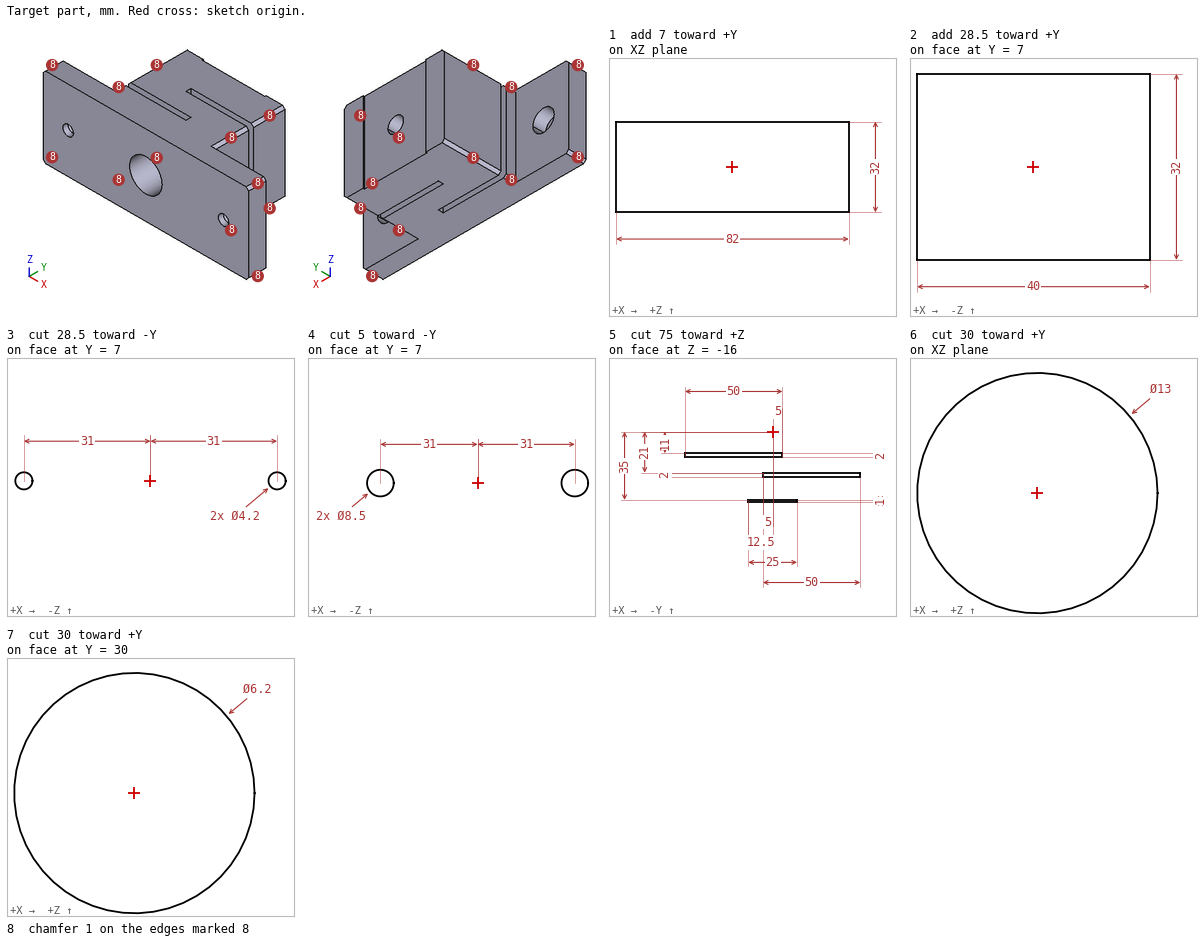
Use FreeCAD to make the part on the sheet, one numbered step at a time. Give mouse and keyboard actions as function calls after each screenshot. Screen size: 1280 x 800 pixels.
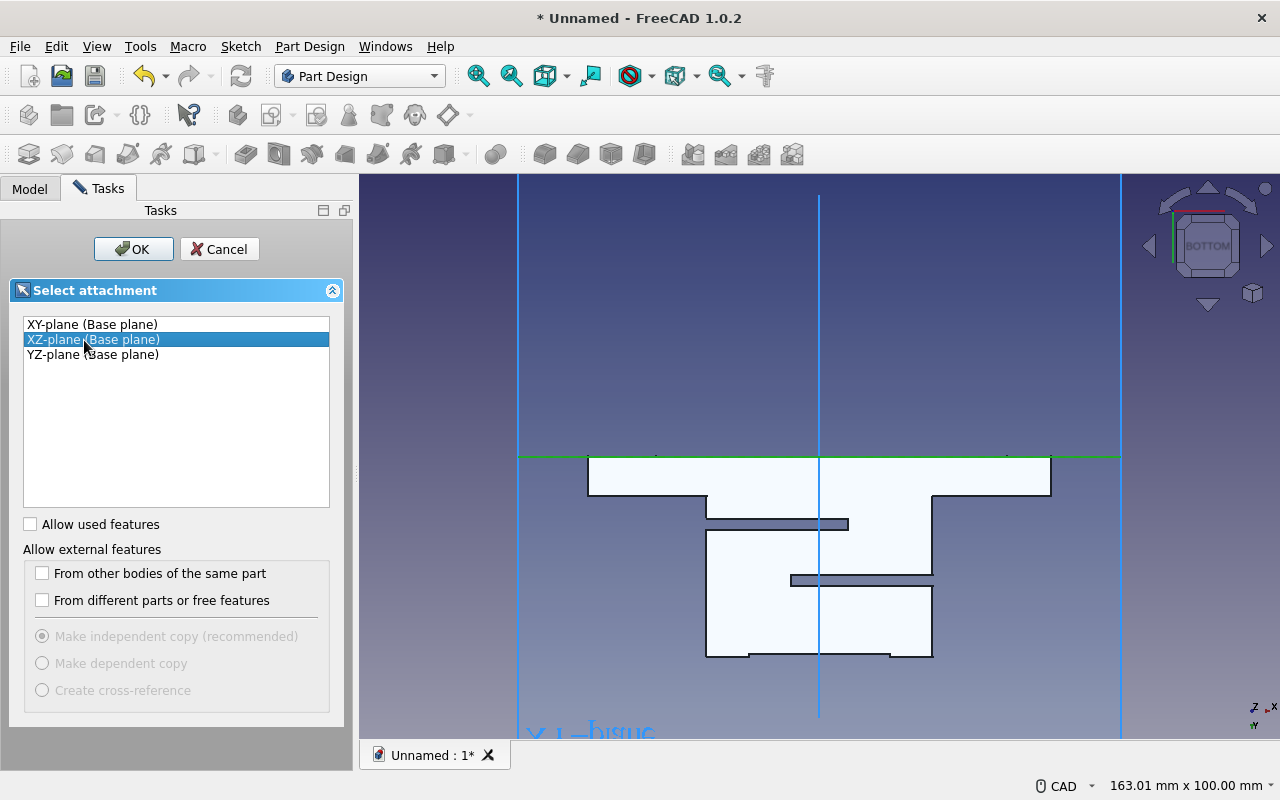
click(134, 249)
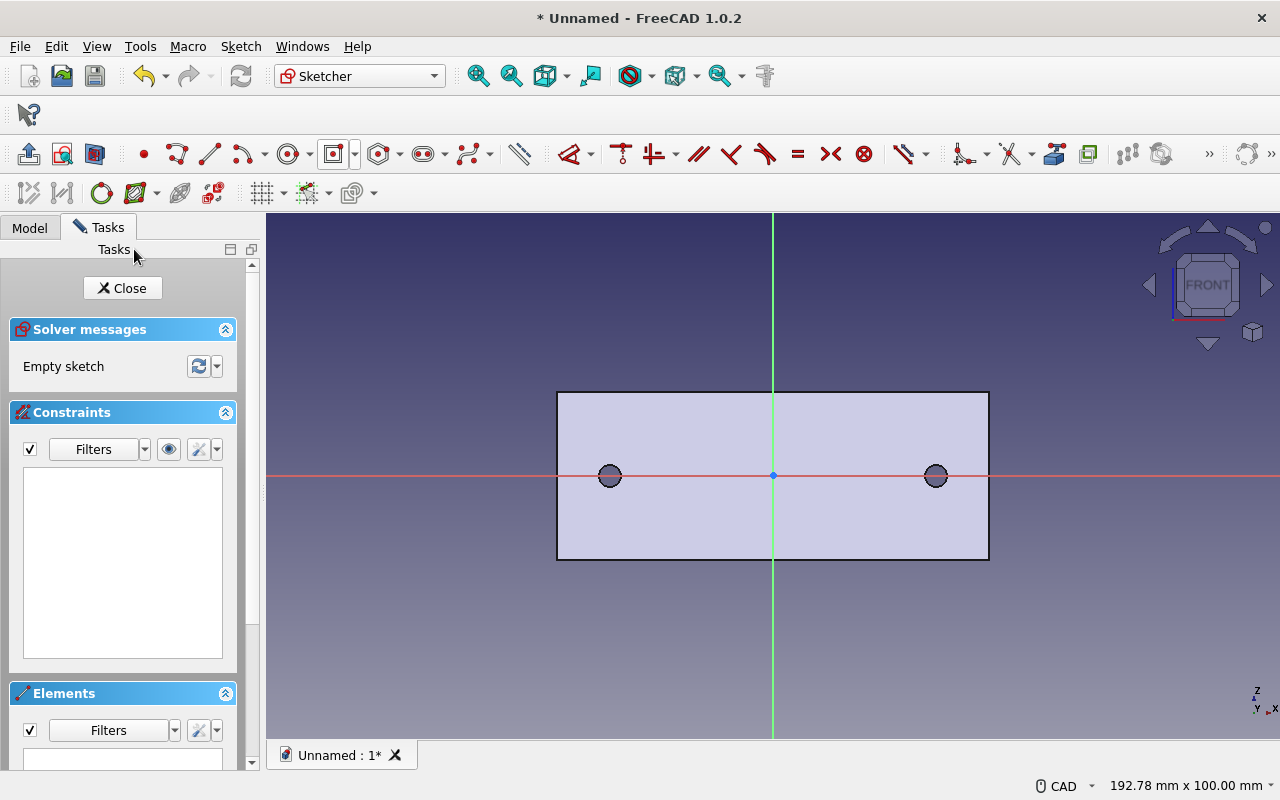
scroll(790, 476, up, 8)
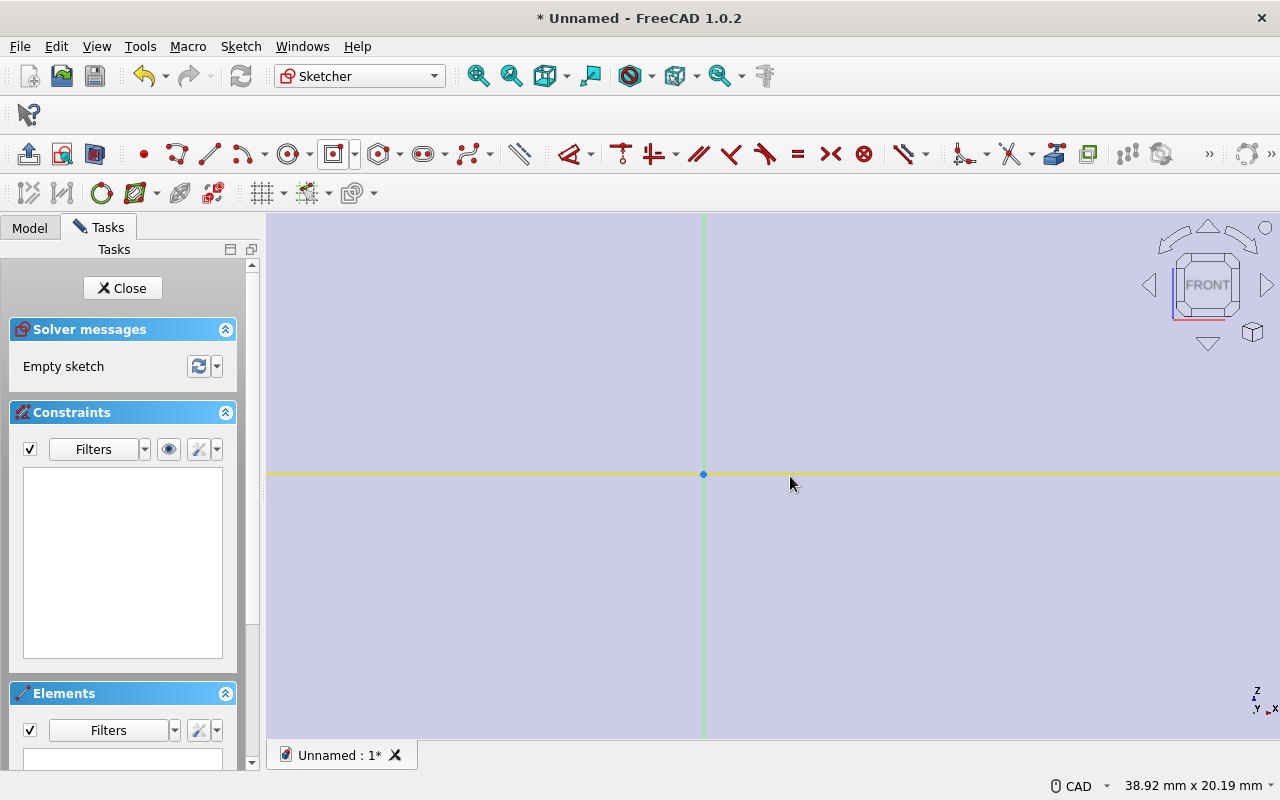
key(g)
key(c)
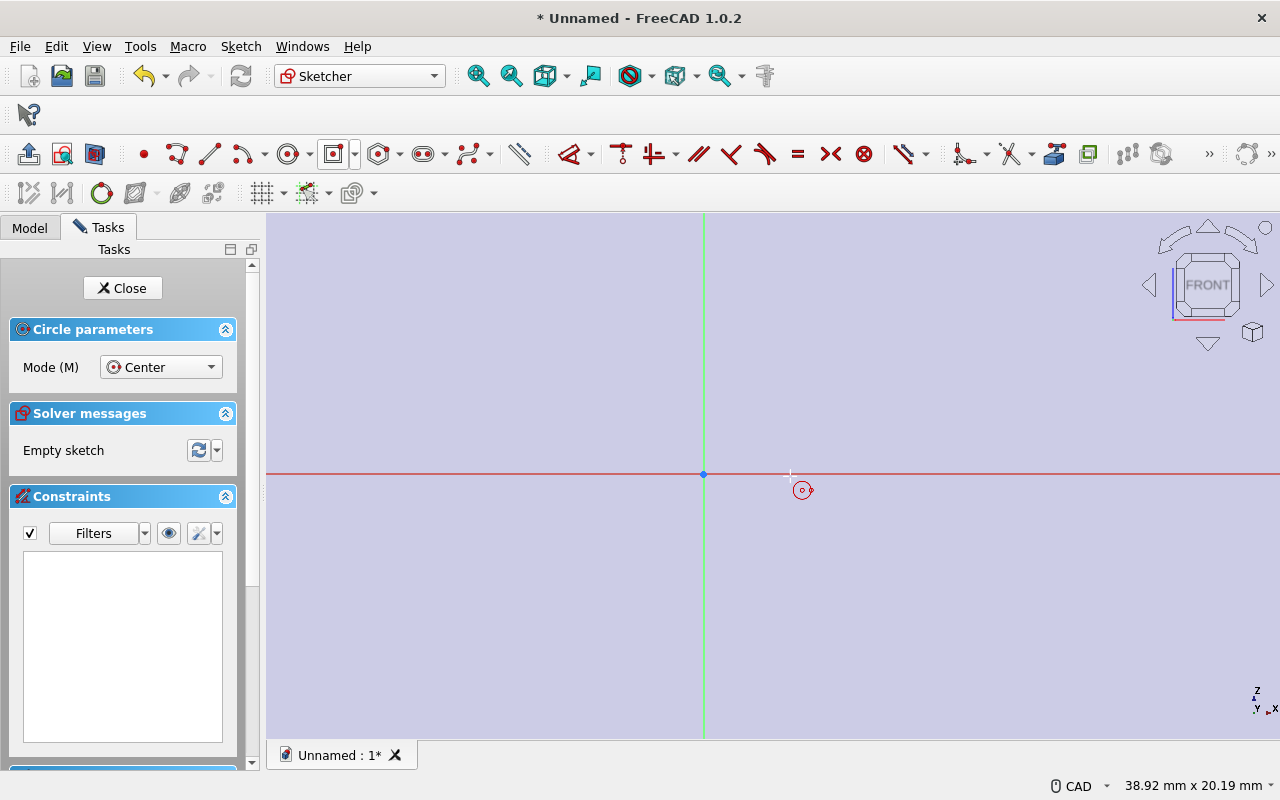
click(704, 474)
move(823, 354)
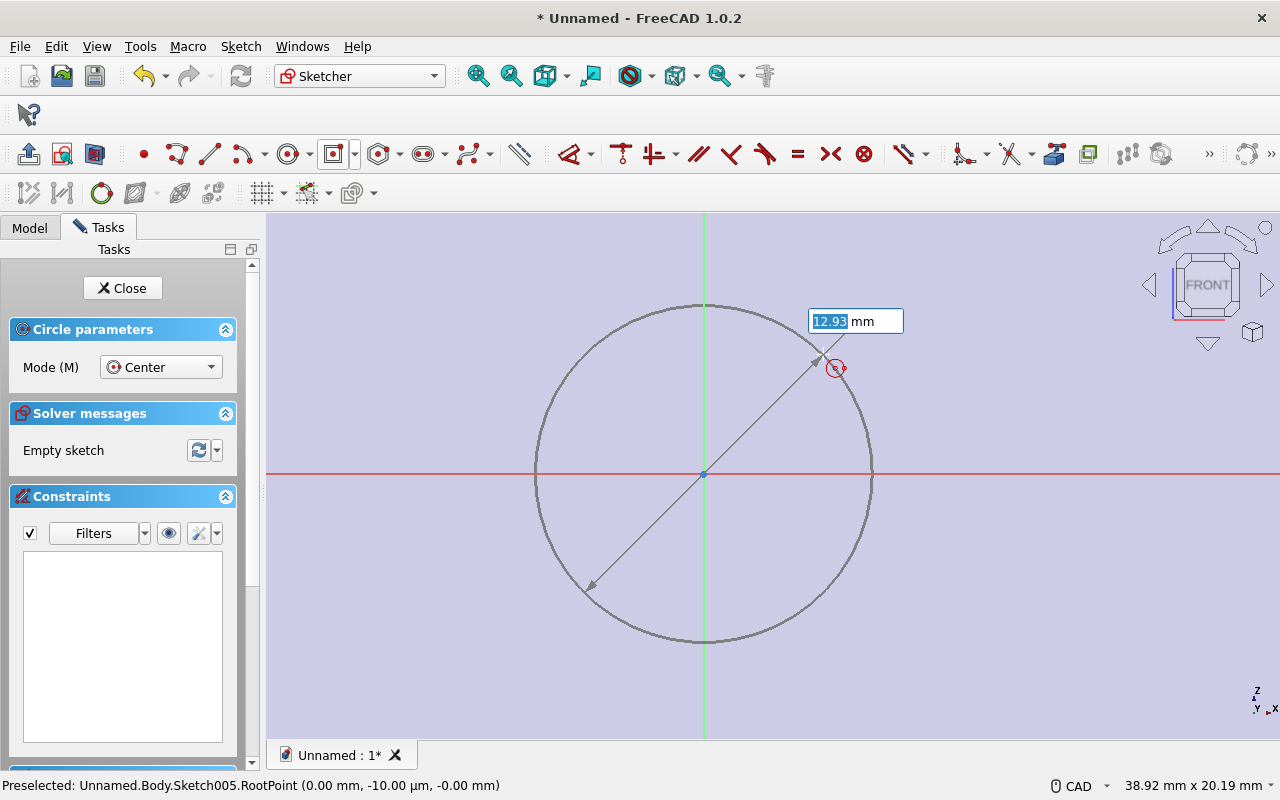
text(13)
key(Return)
key(Escape)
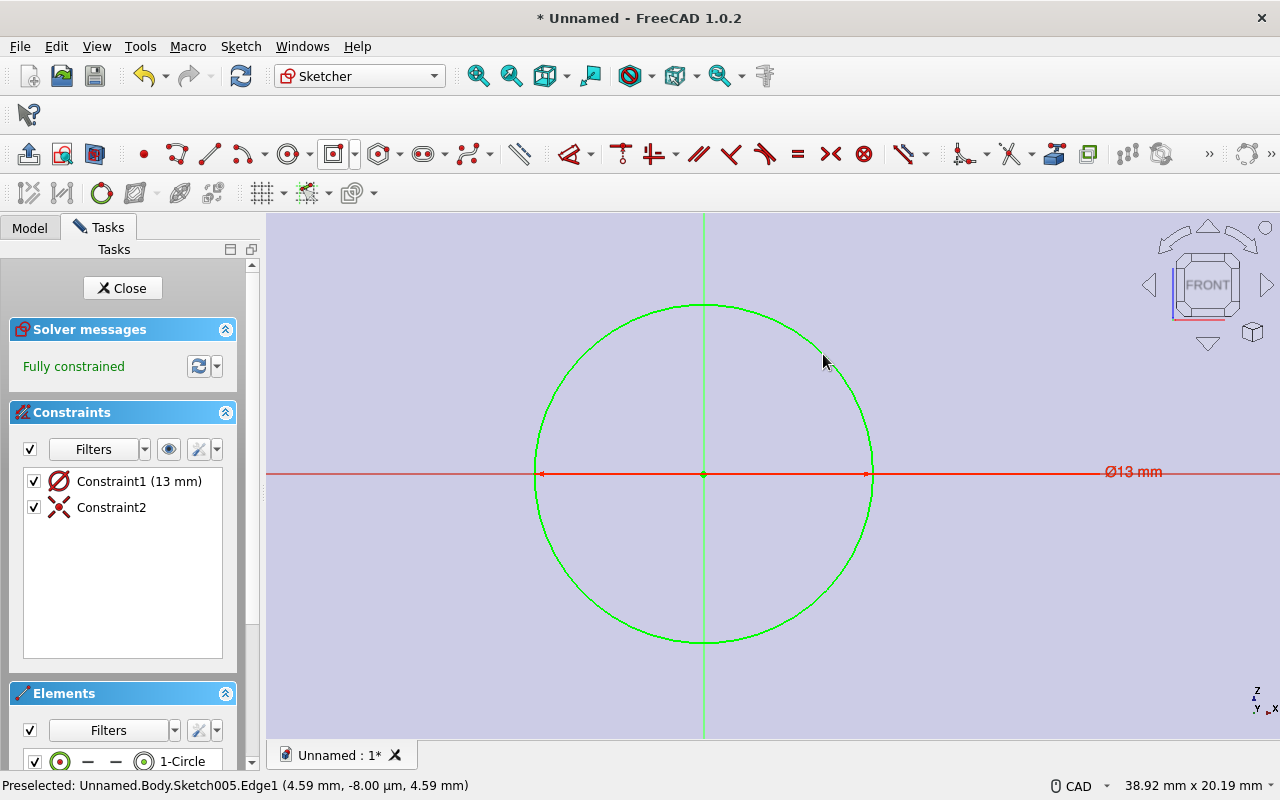
click(123, 288)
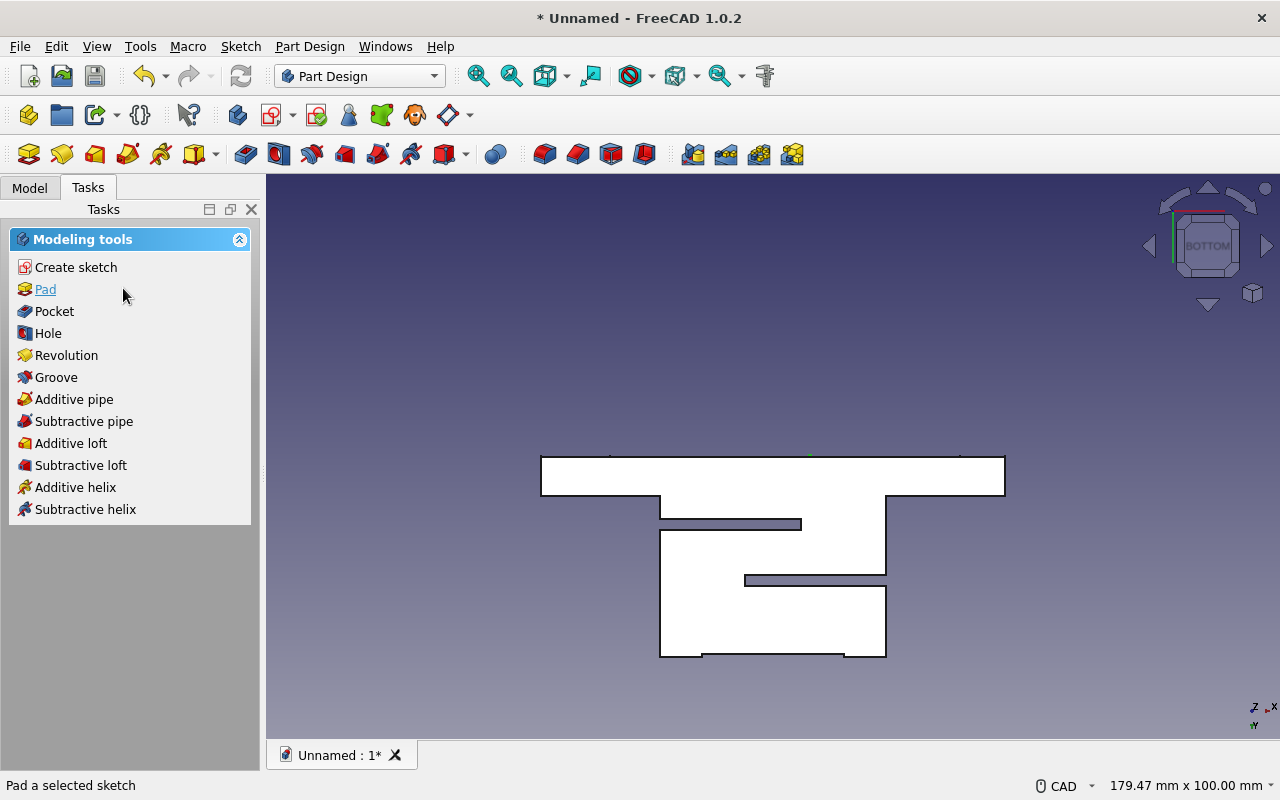
click(246, 154)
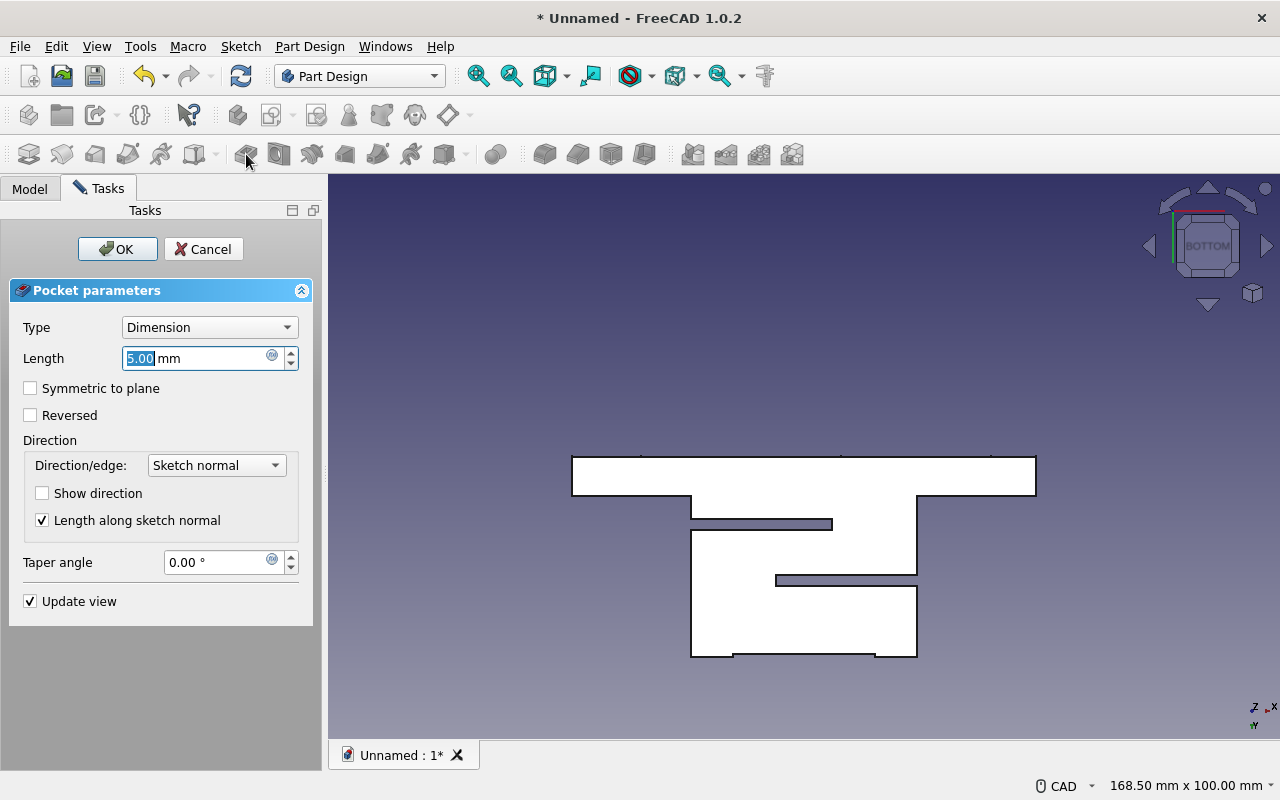
text(30)
key(Tab)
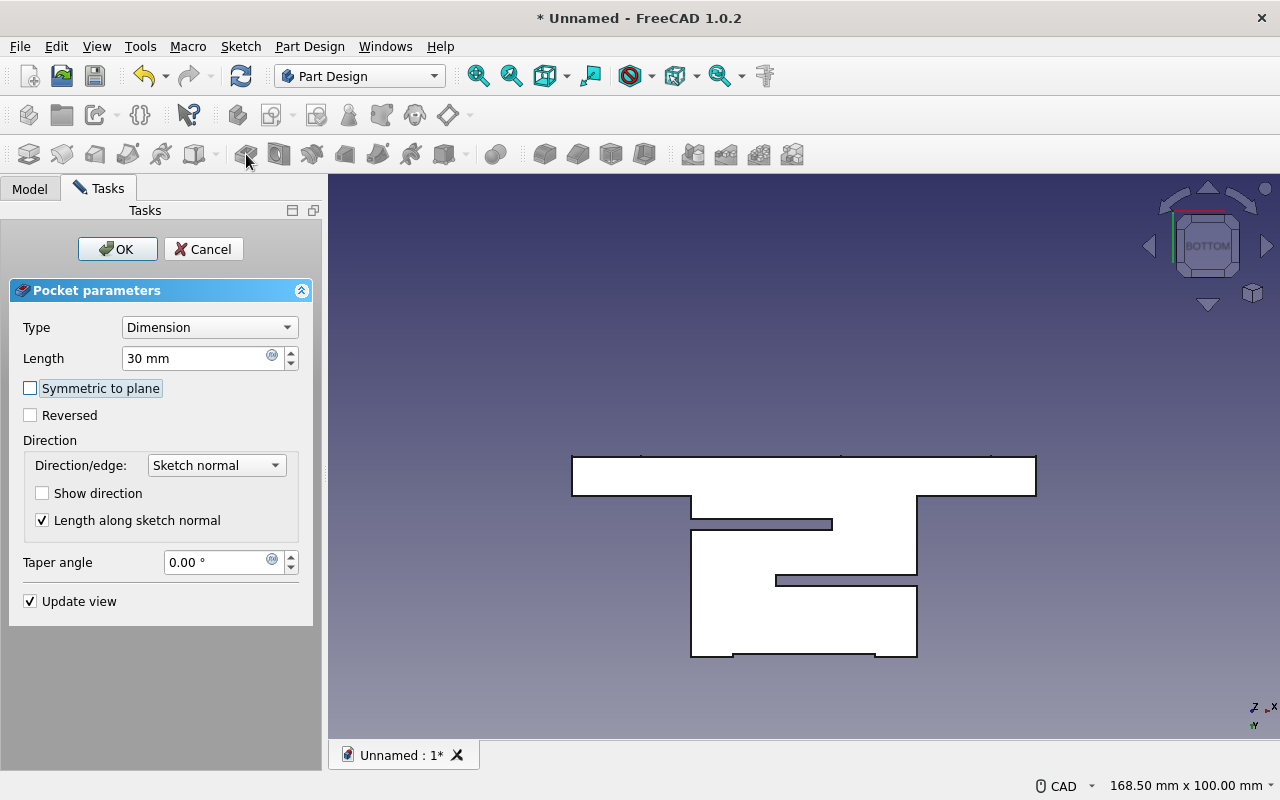
click(118, 249)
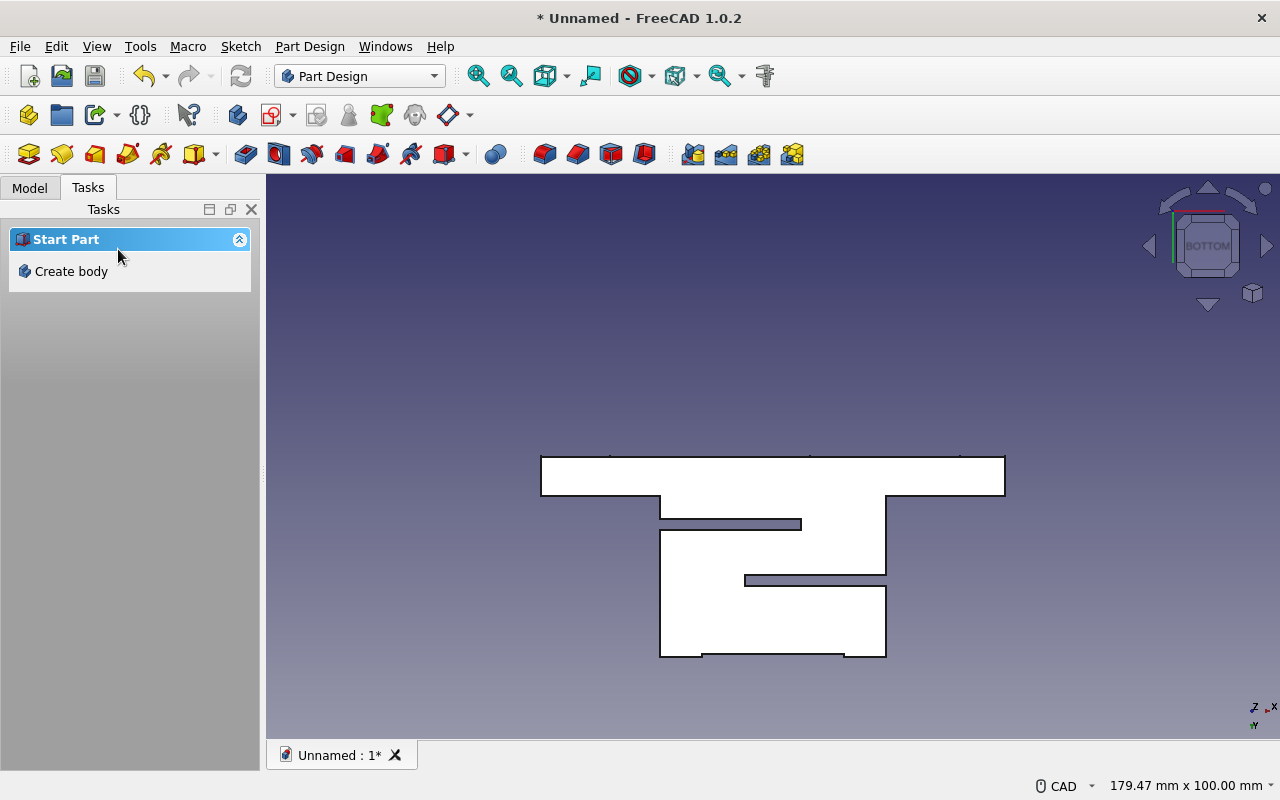
key(0)